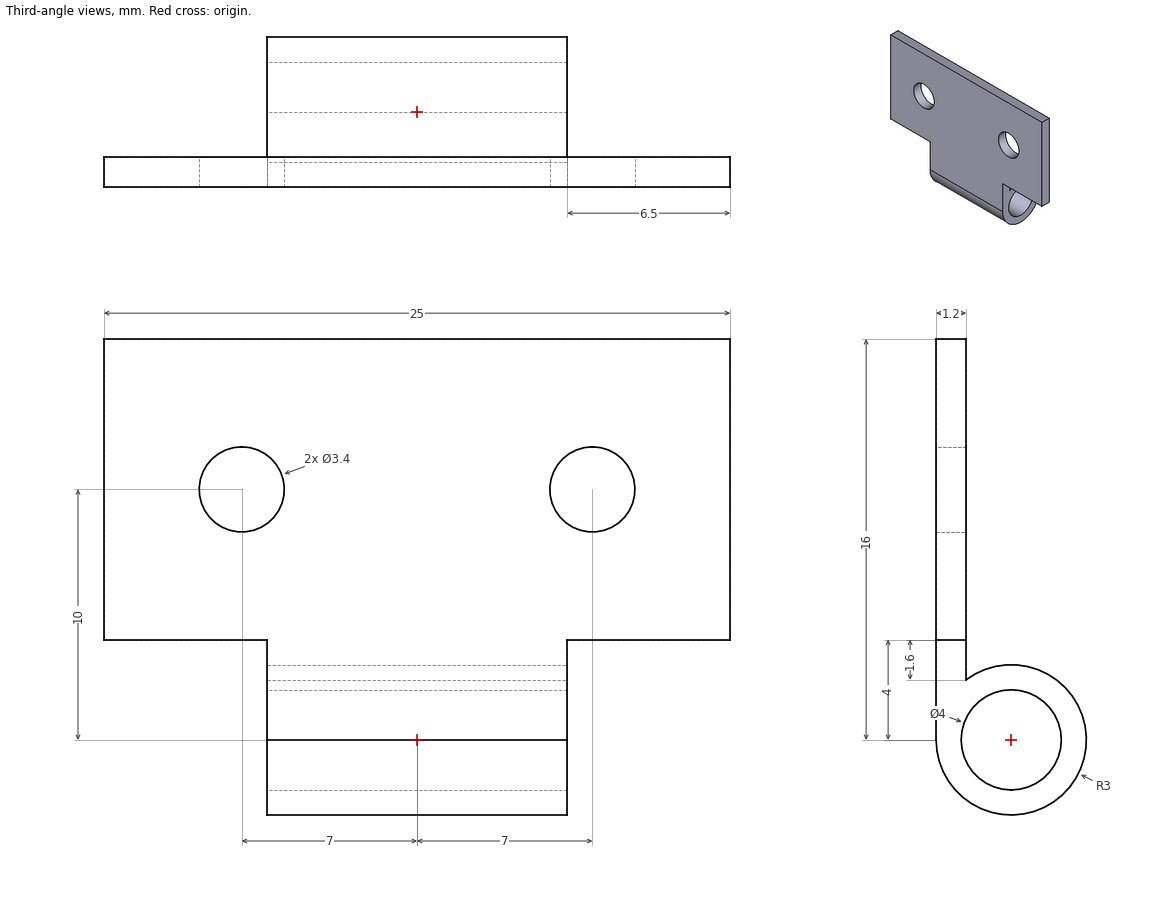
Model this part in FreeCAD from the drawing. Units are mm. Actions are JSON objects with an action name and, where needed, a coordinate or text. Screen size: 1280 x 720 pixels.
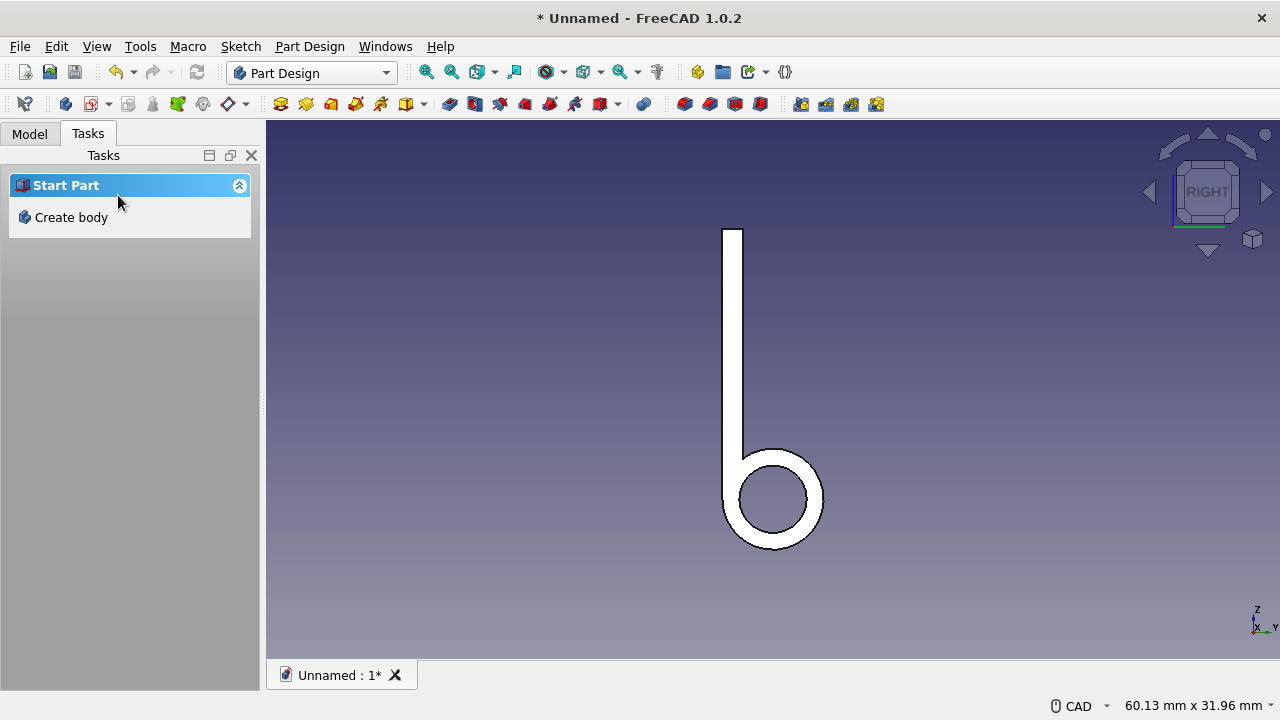
{"action": "key", "text": "2"}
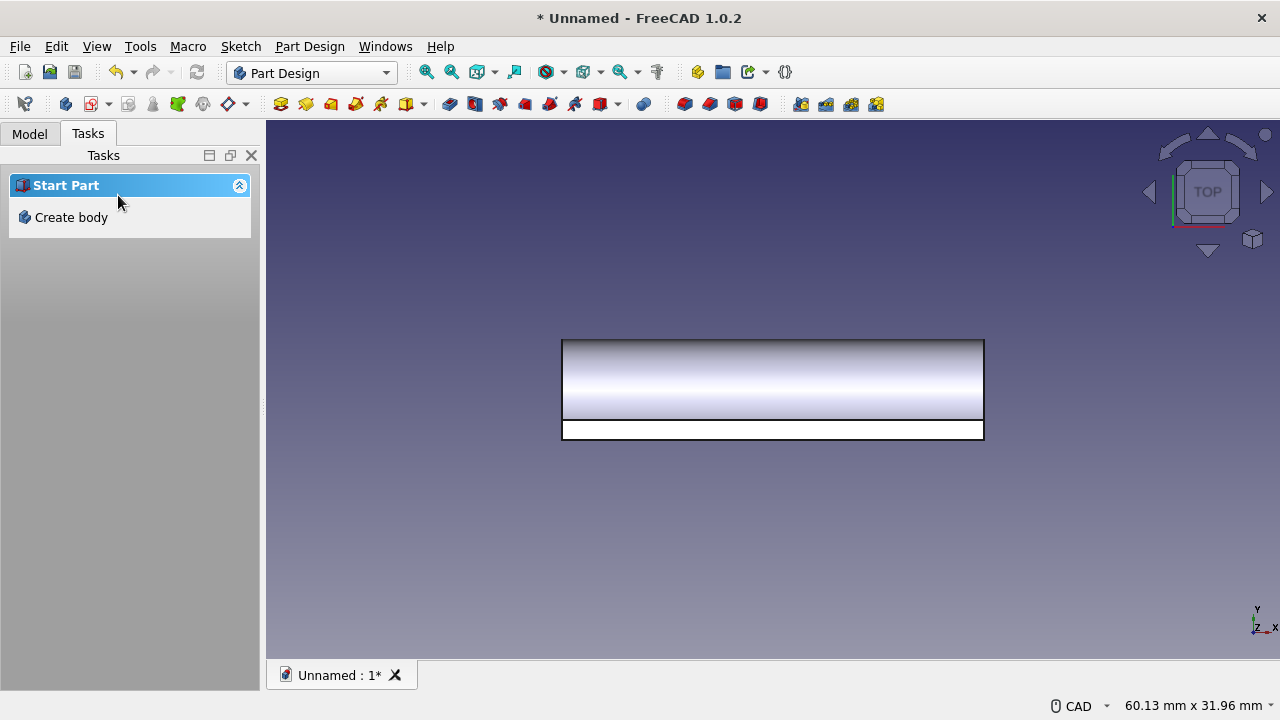
{"action": "left_click", "coordinate": [427, 72]}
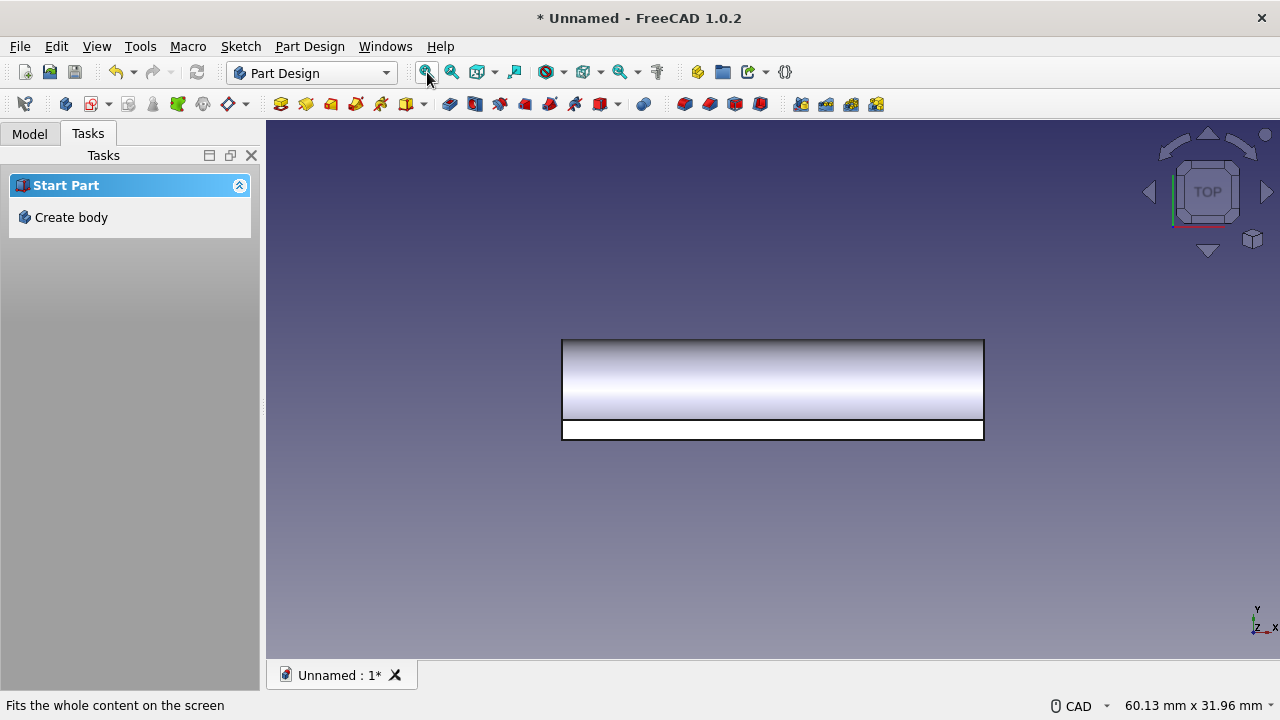
{"action": "left_click", "coordinate": [30, 134]}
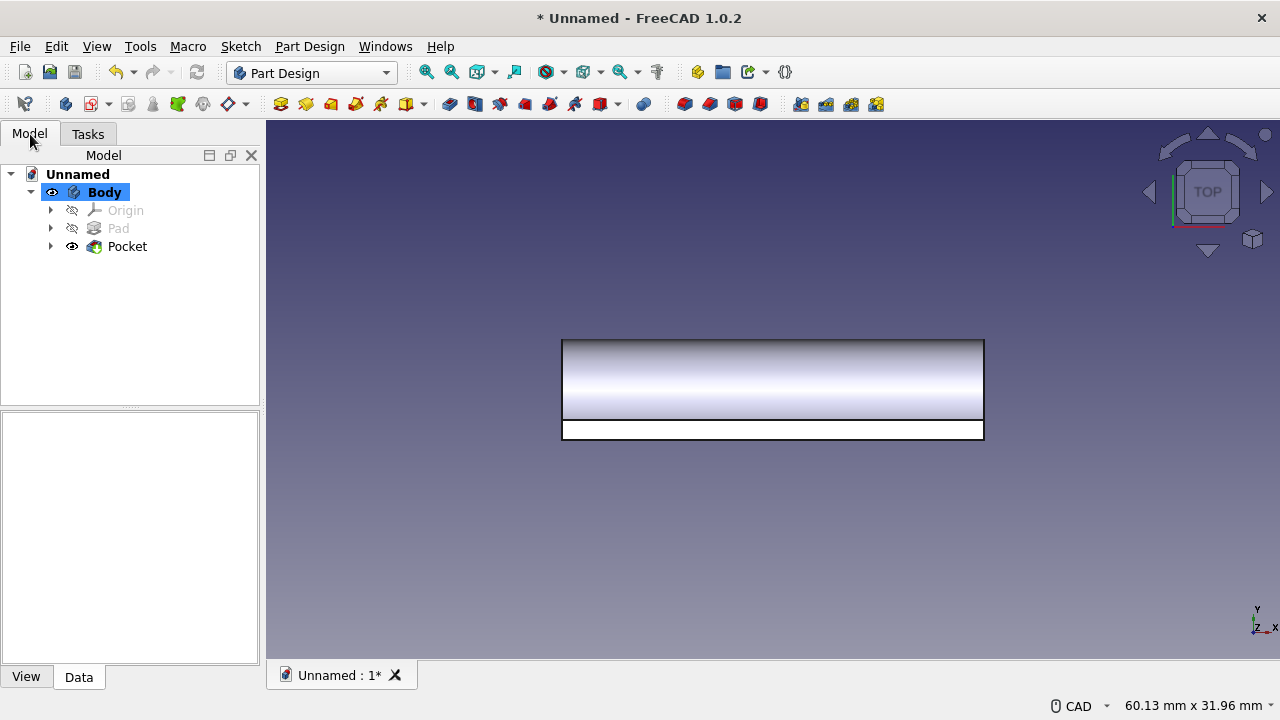
{"action": "left_click", "coordinate": [51, 210]}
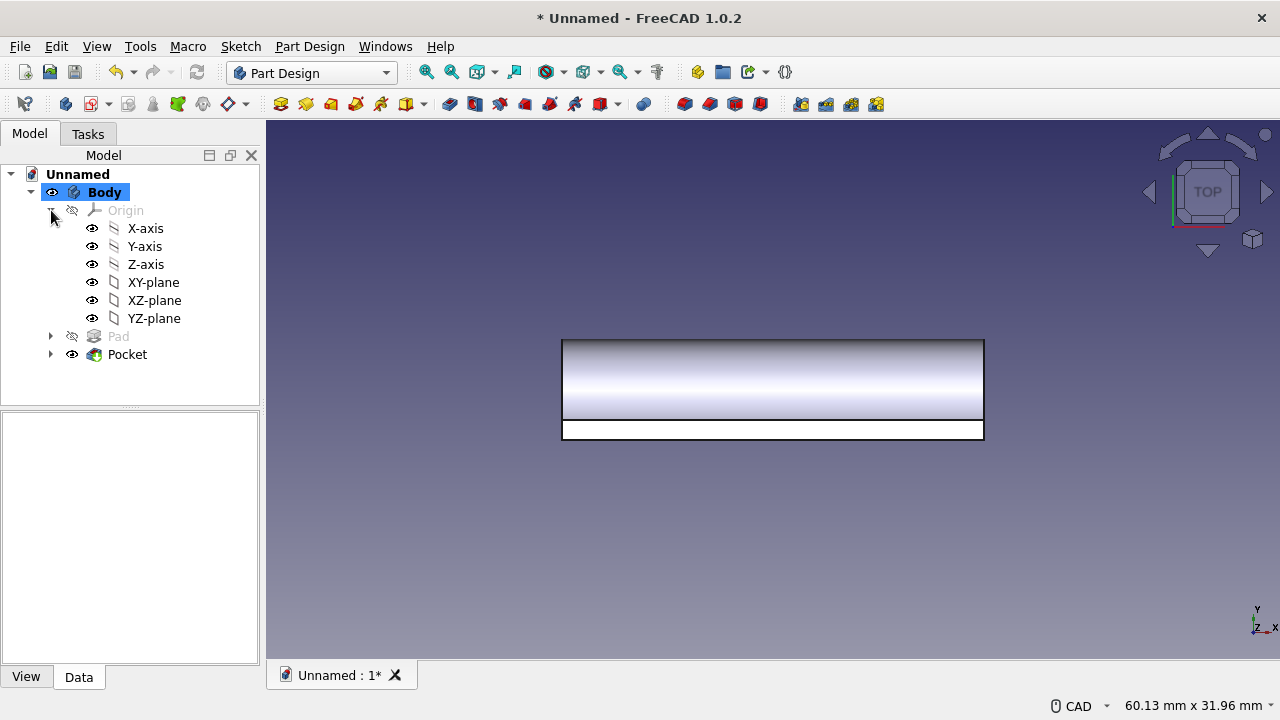
{"action": "left_click", "coordinate": [137, 318]}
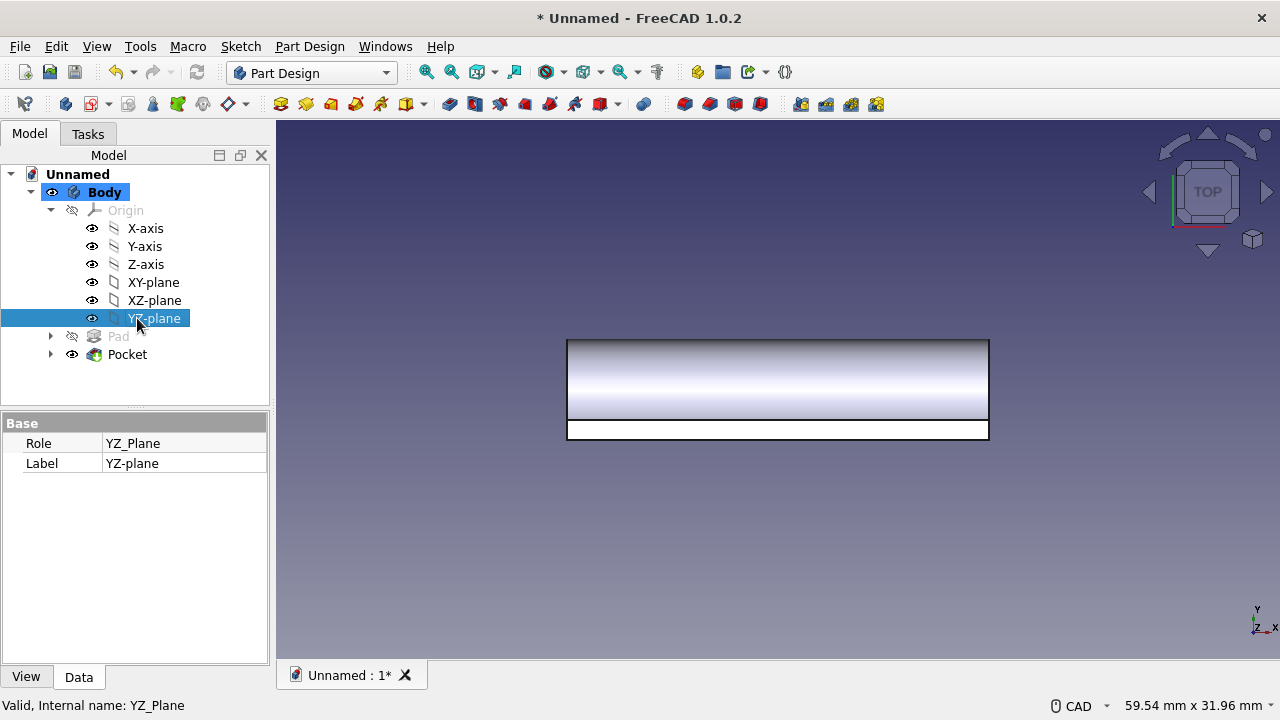
{"action": "left_click", "coordinate": [228, 104]}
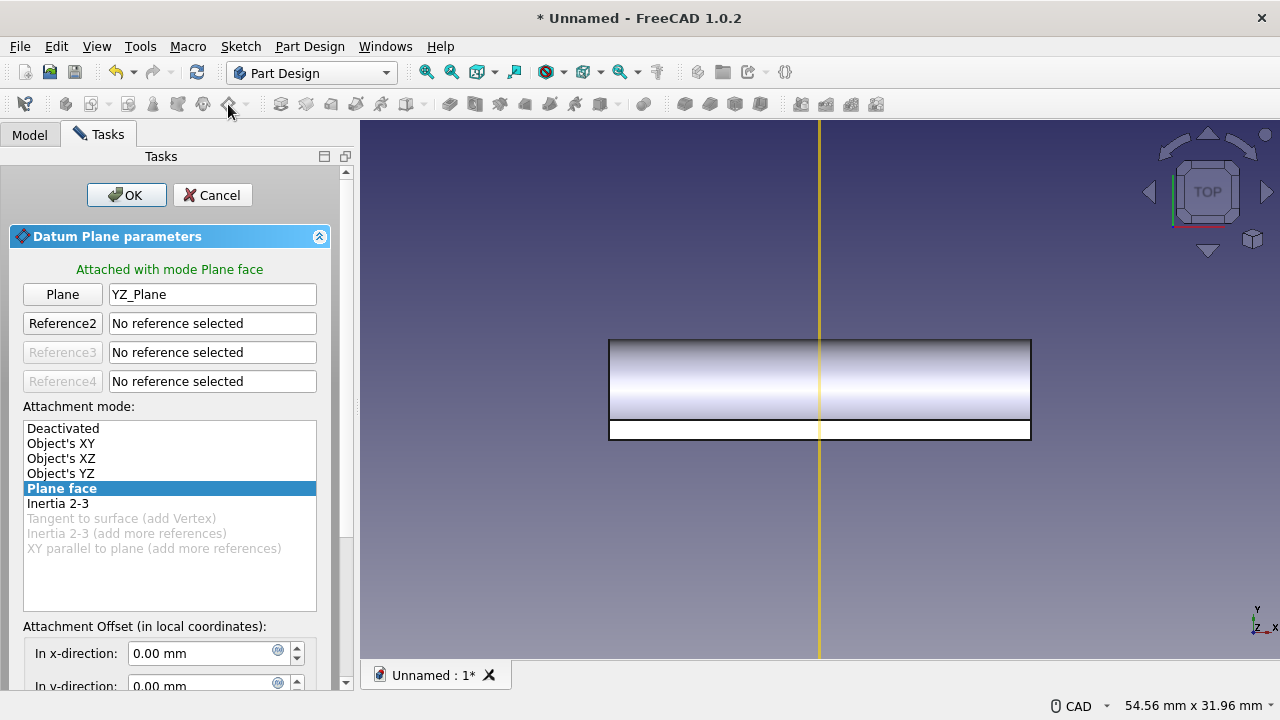
{"action": "scroll", "coordinate": [346, 428], "scroll_direction": "down", "scroll_amount": 2}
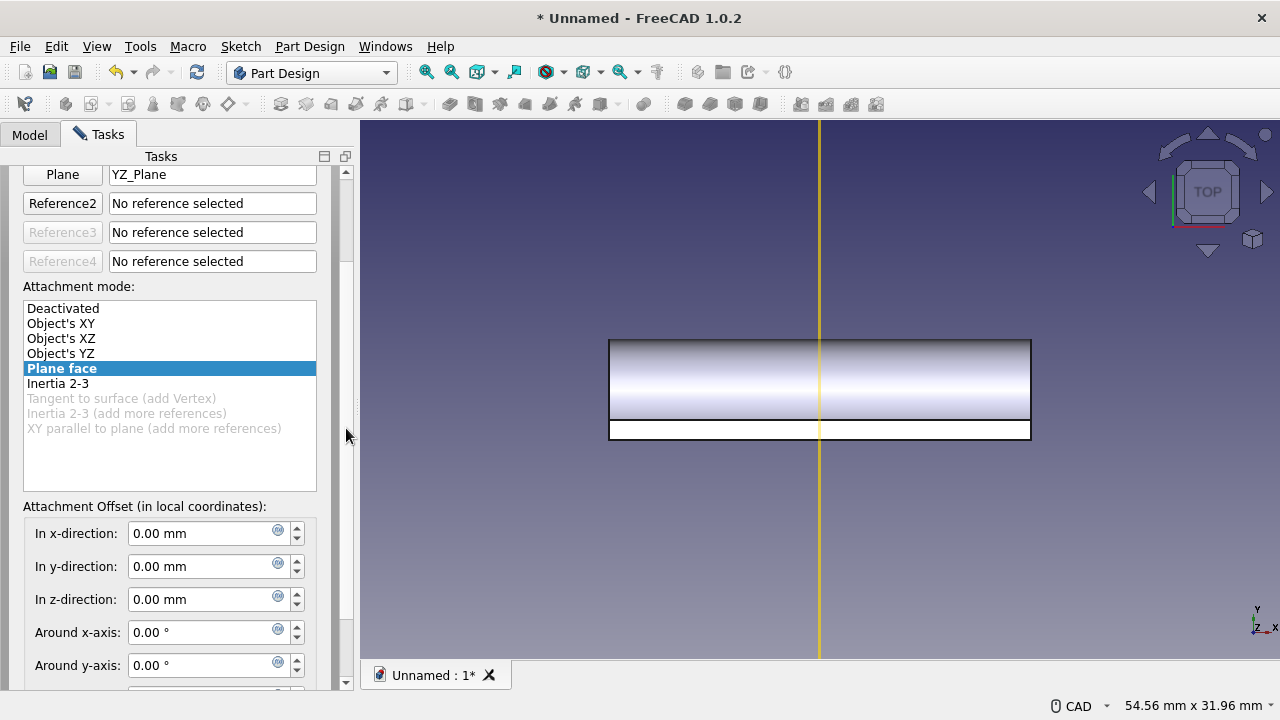
{"action": "triple_click", "coordinate": [210, 600]}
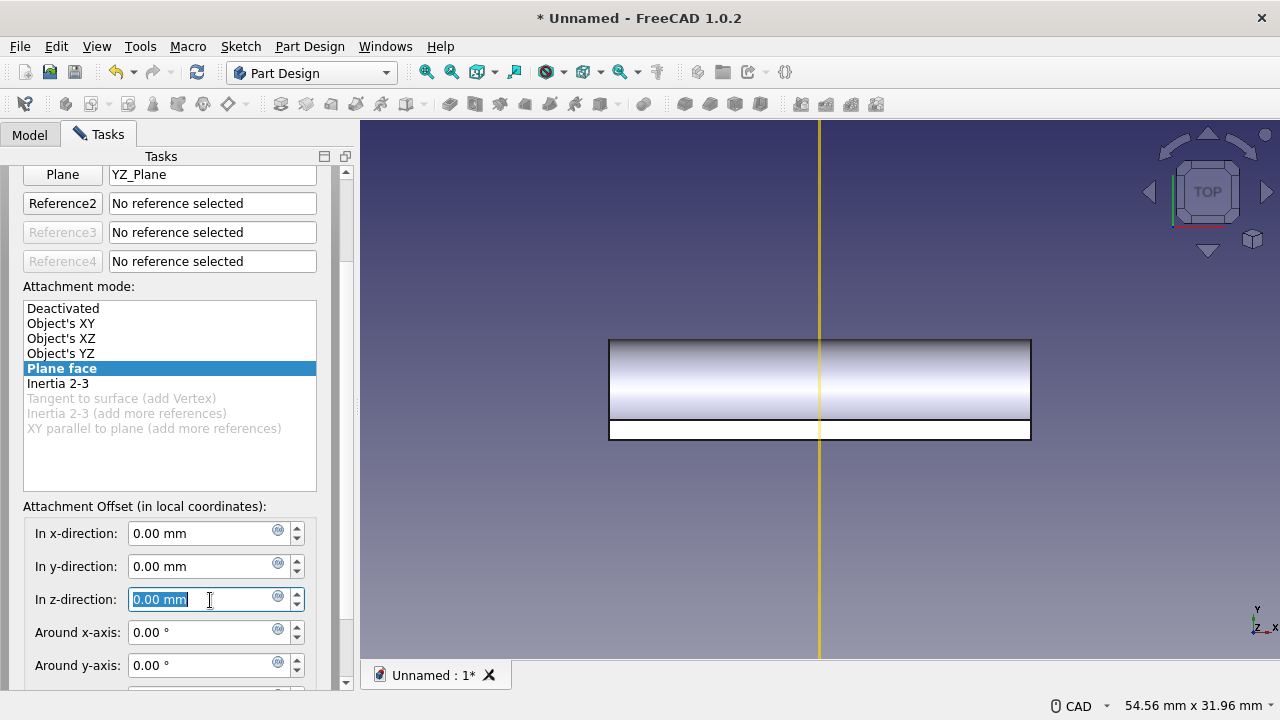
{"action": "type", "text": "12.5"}
{"action": "key", "text": "Tab"}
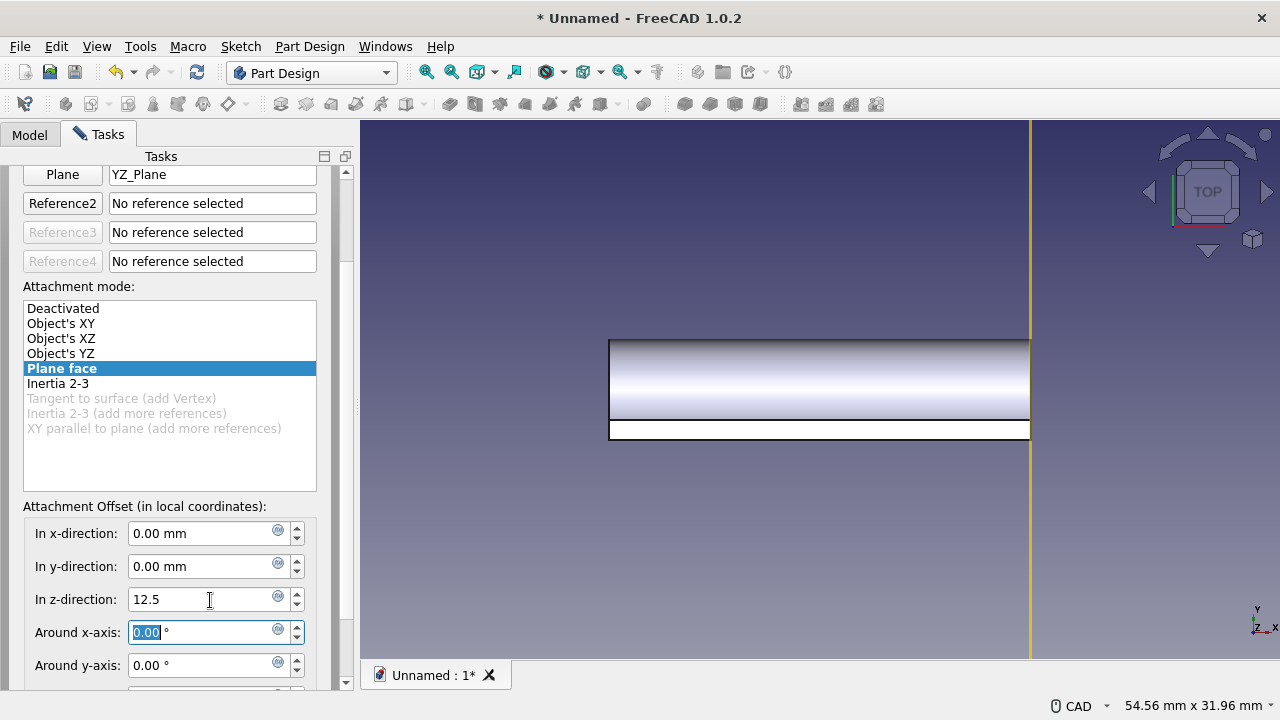
{"action": "scroll", "coordinate": [346, 428], "scroll_direction": "up", "scroll_amount": 3}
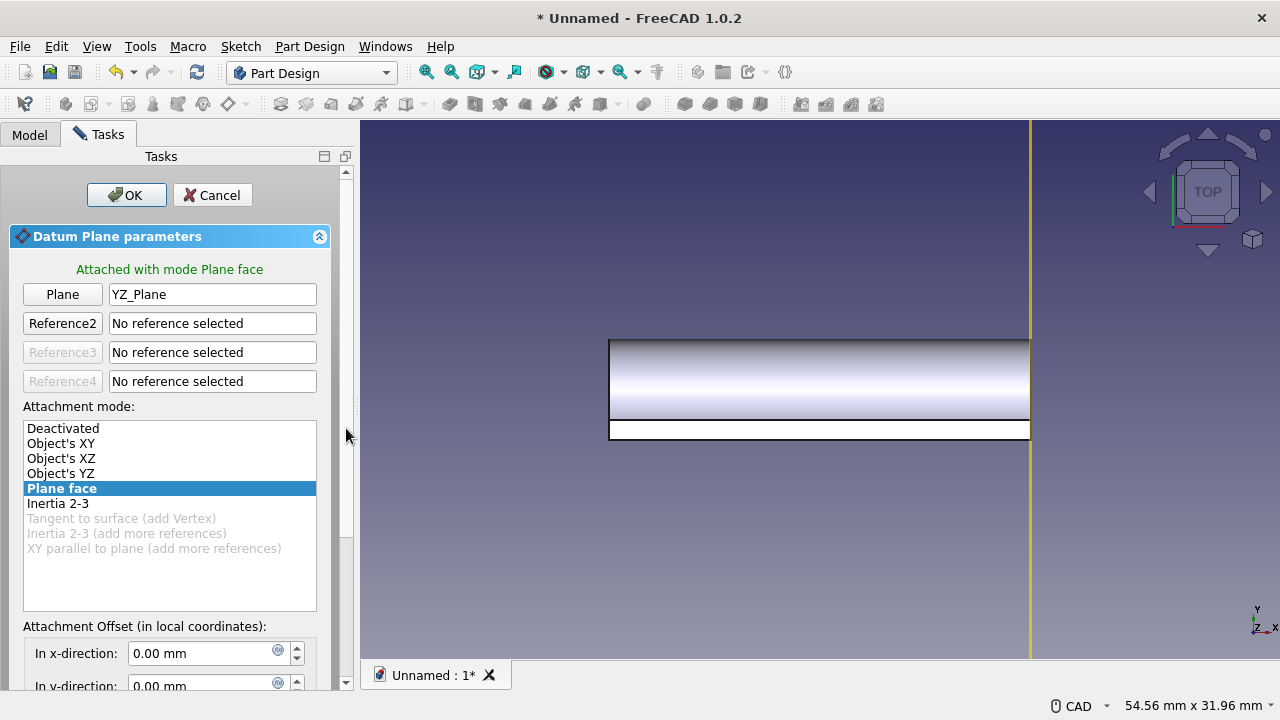
{"action": "left_click", "coordinate": [127, 195]}